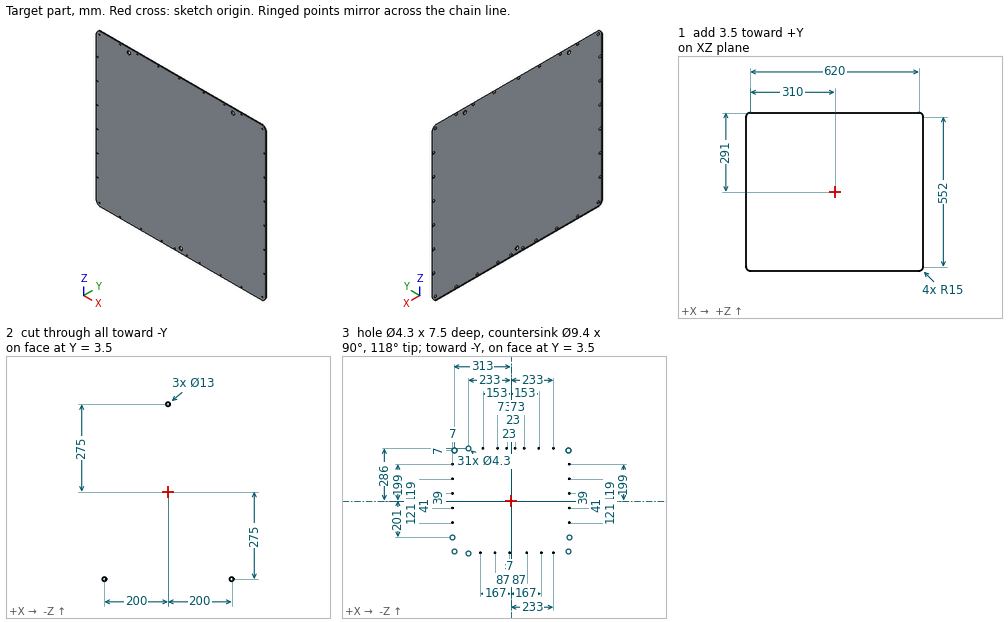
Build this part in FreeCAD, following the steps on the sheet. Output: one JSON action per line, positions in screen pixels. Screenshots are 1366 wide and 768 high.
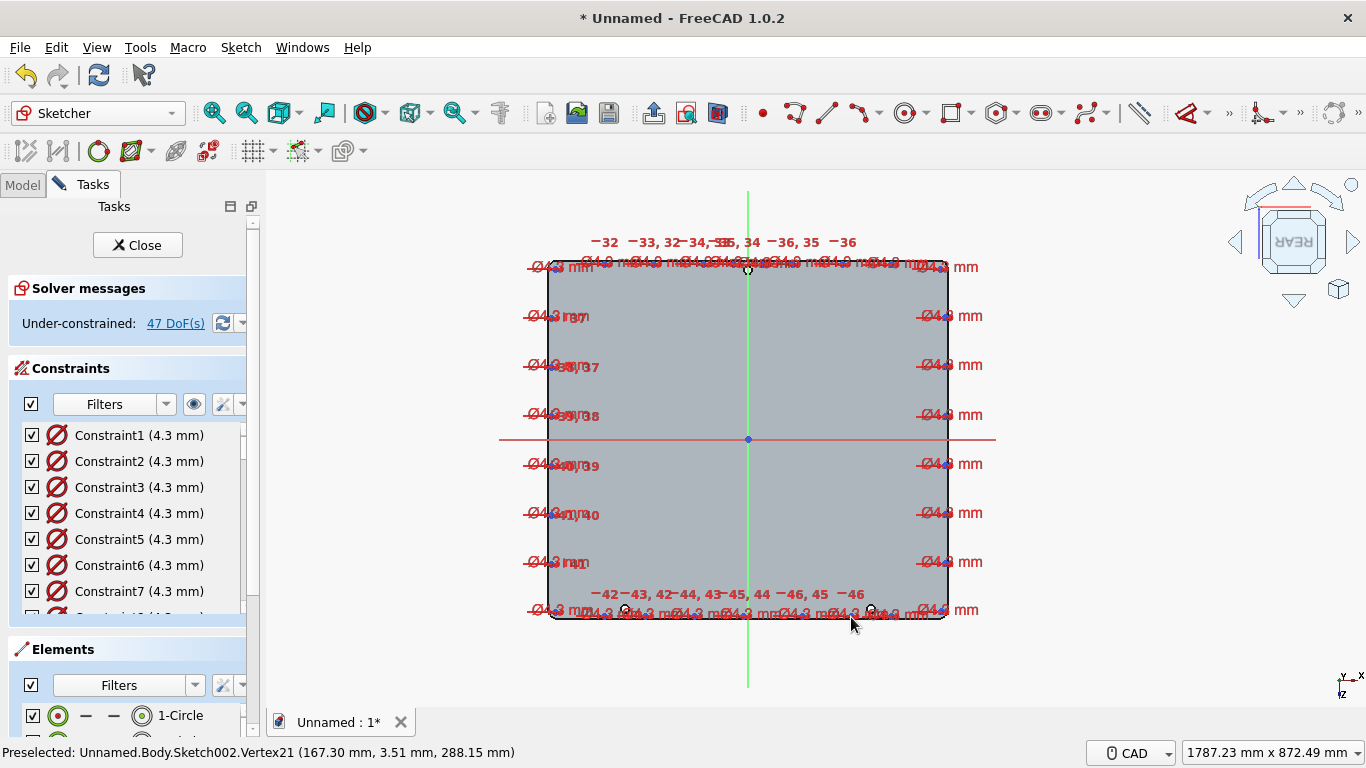
{"action": "left_click", "coordinate": [945, 564]}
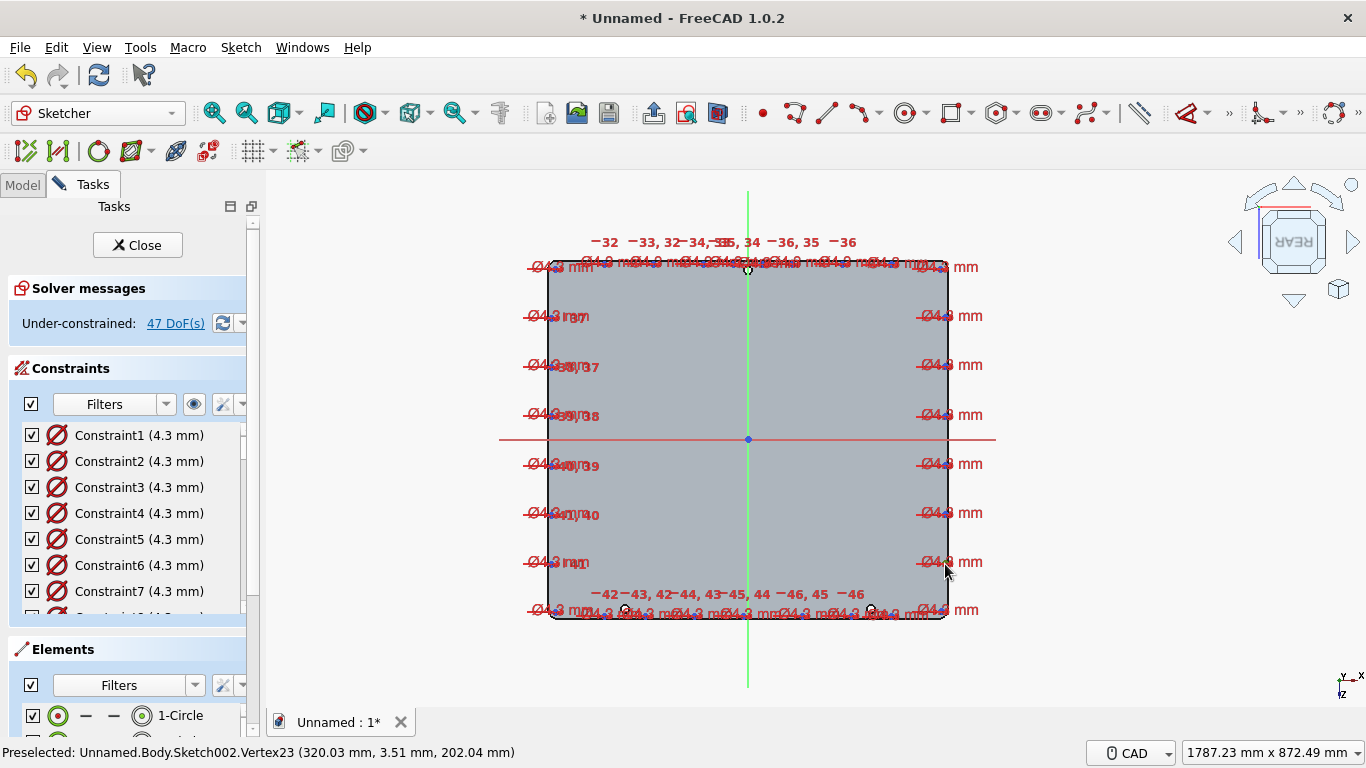
{"action": "left_click", "coordinate": [945, 515]}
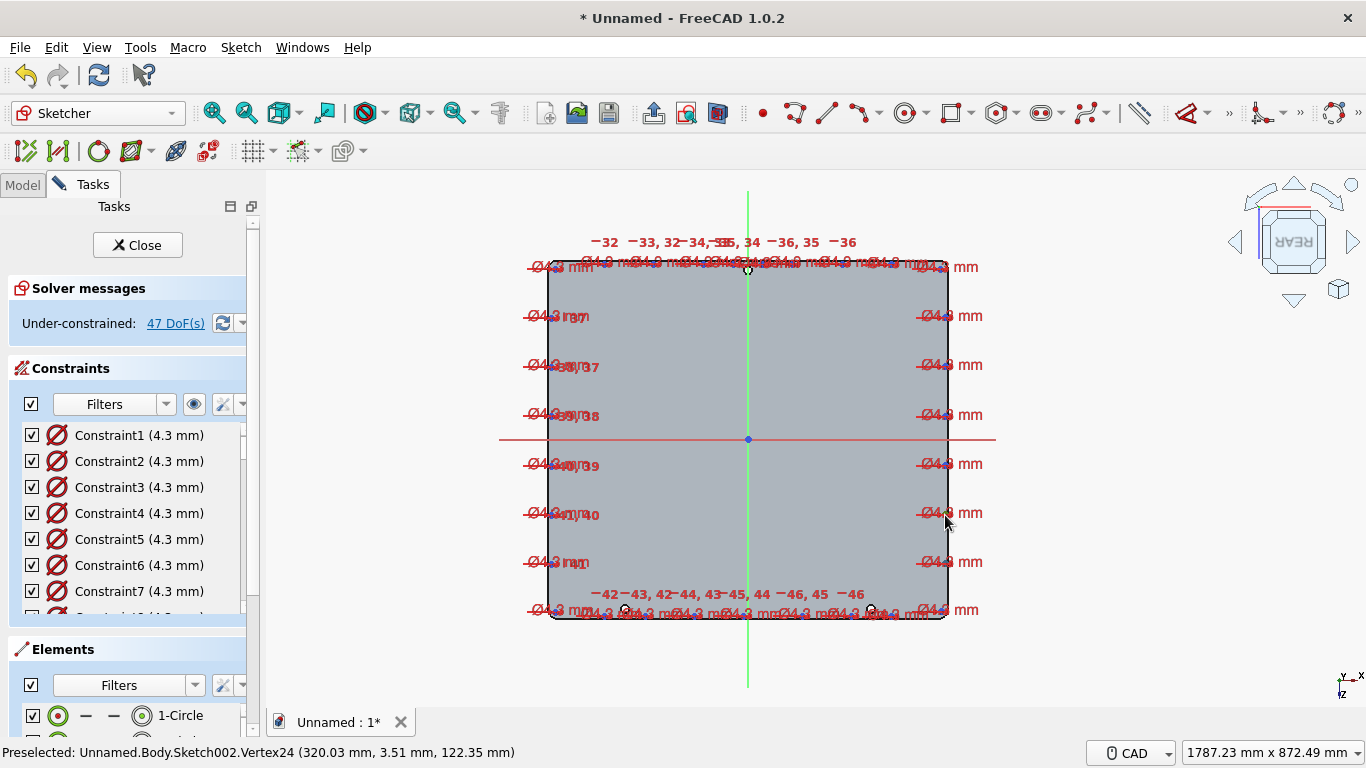
{"action": "key", "text": "v"}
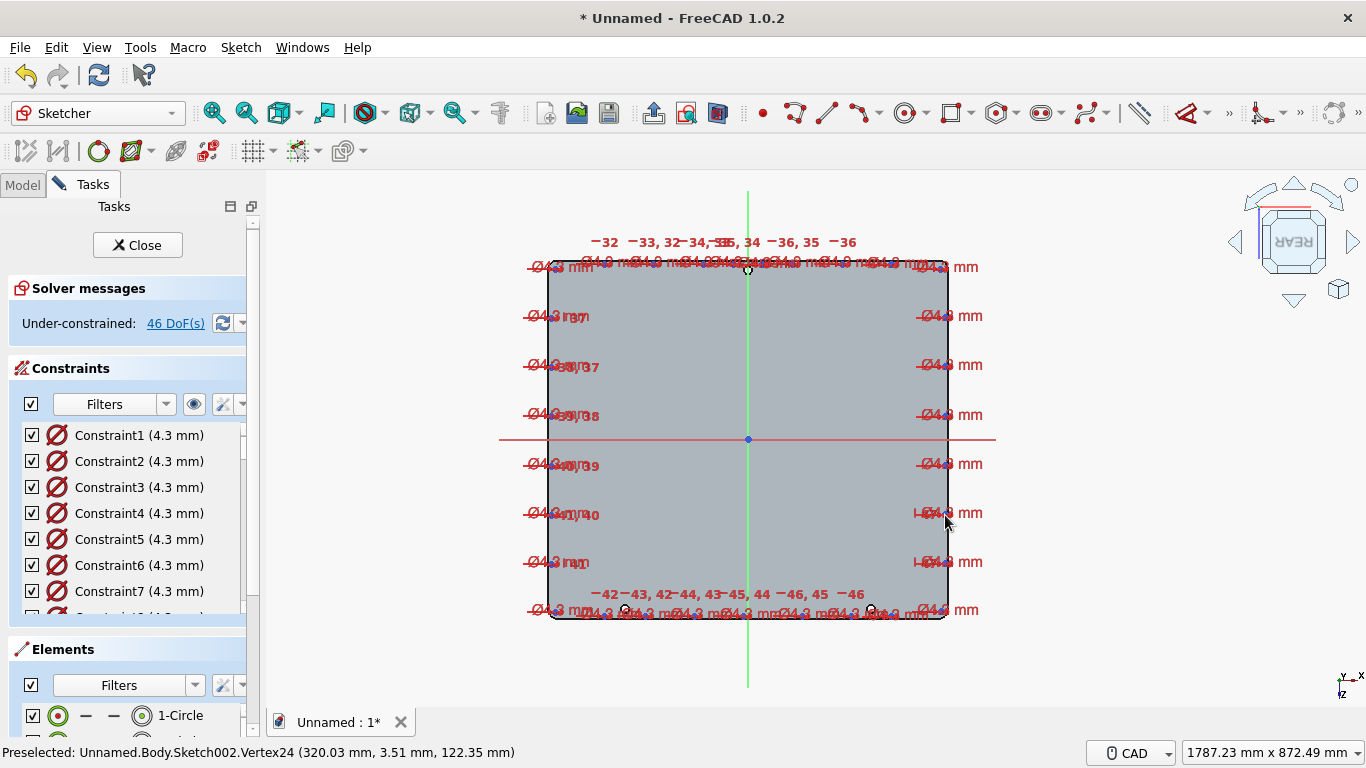
{"action": "left_click", "coordinate": [945, 515]}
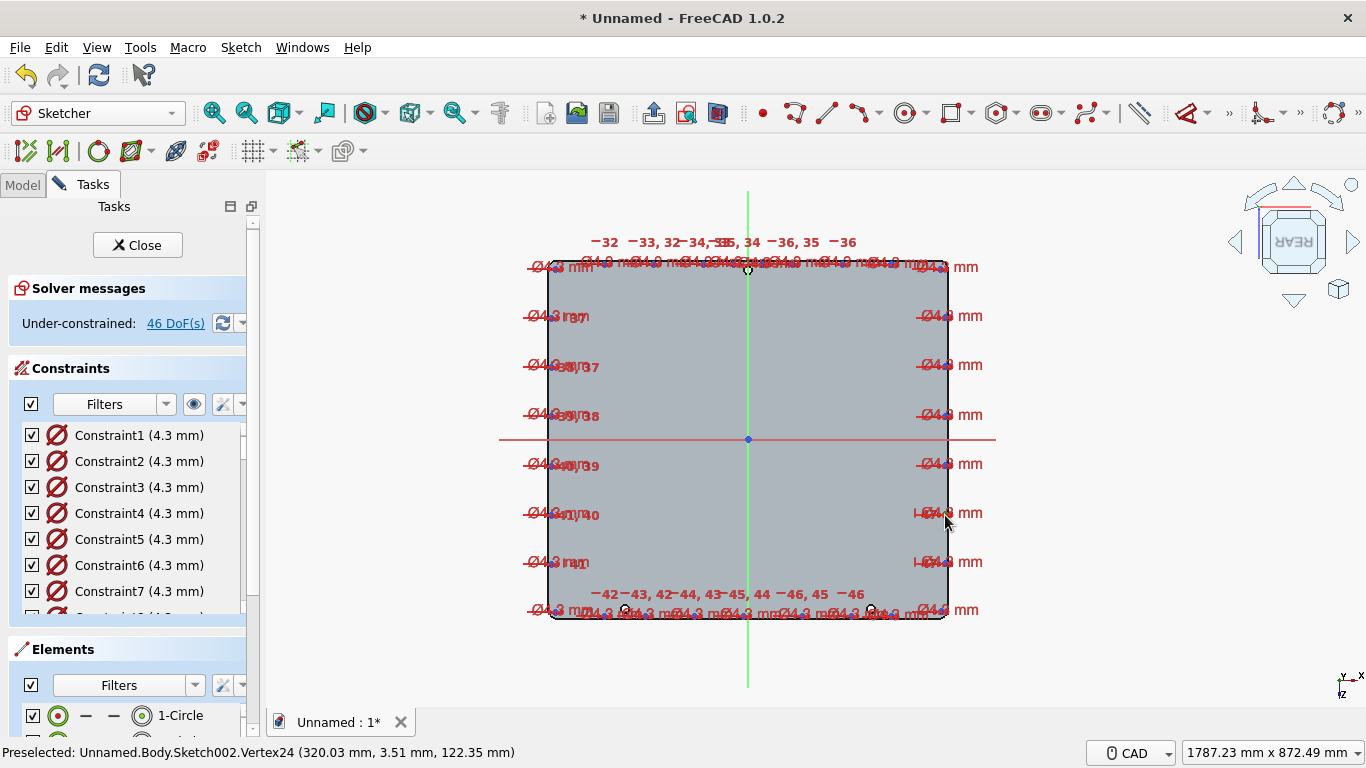
{"action": "left_click", "coordinate": [945, 466]}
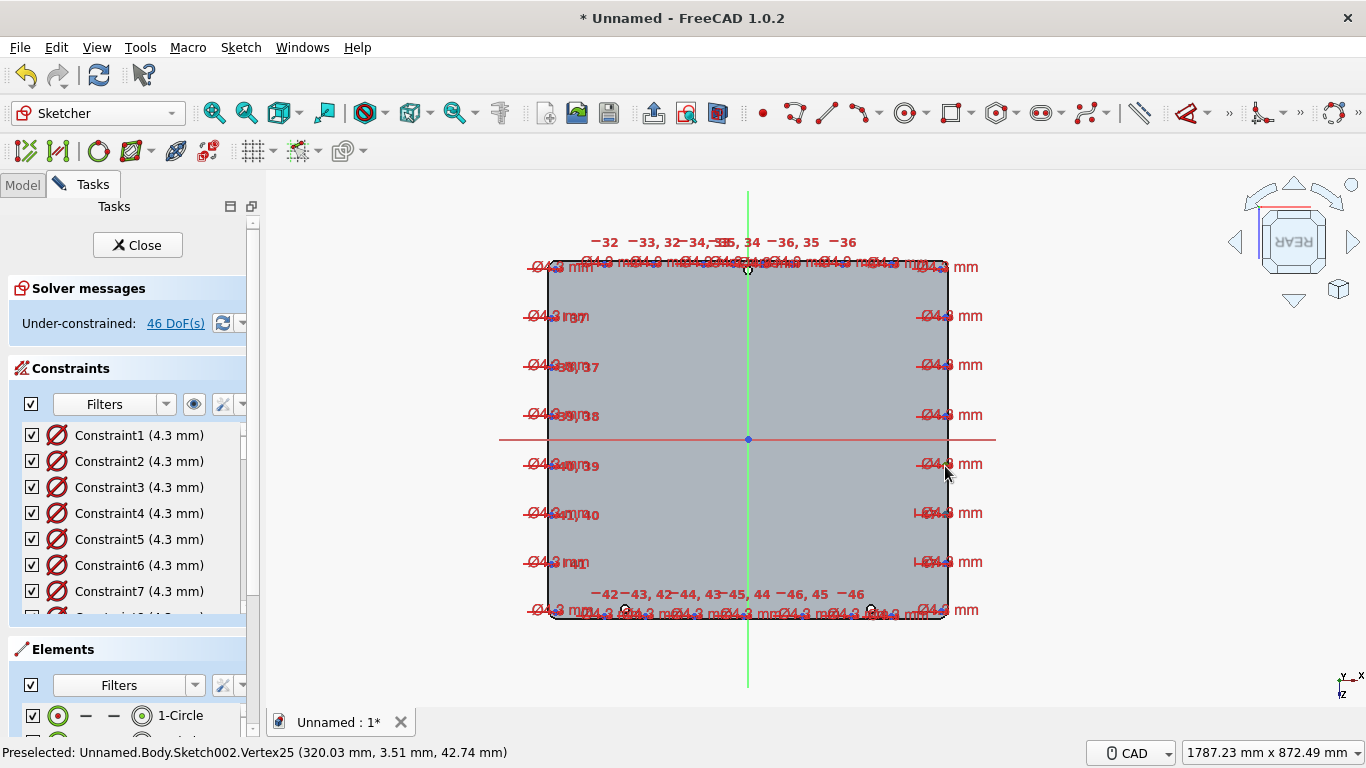
{"action": "key", "text": "v"}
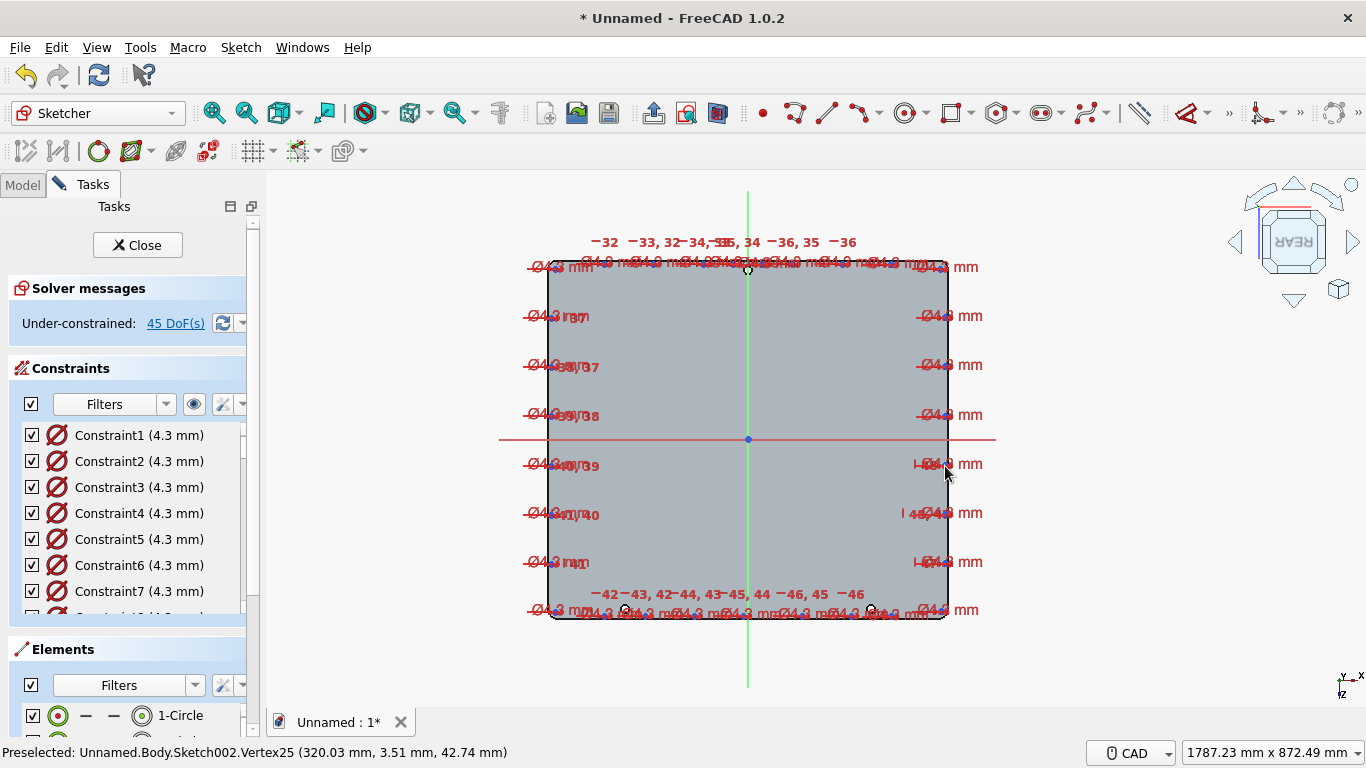
{"action": "left_click", "coordinate": [945, 466]}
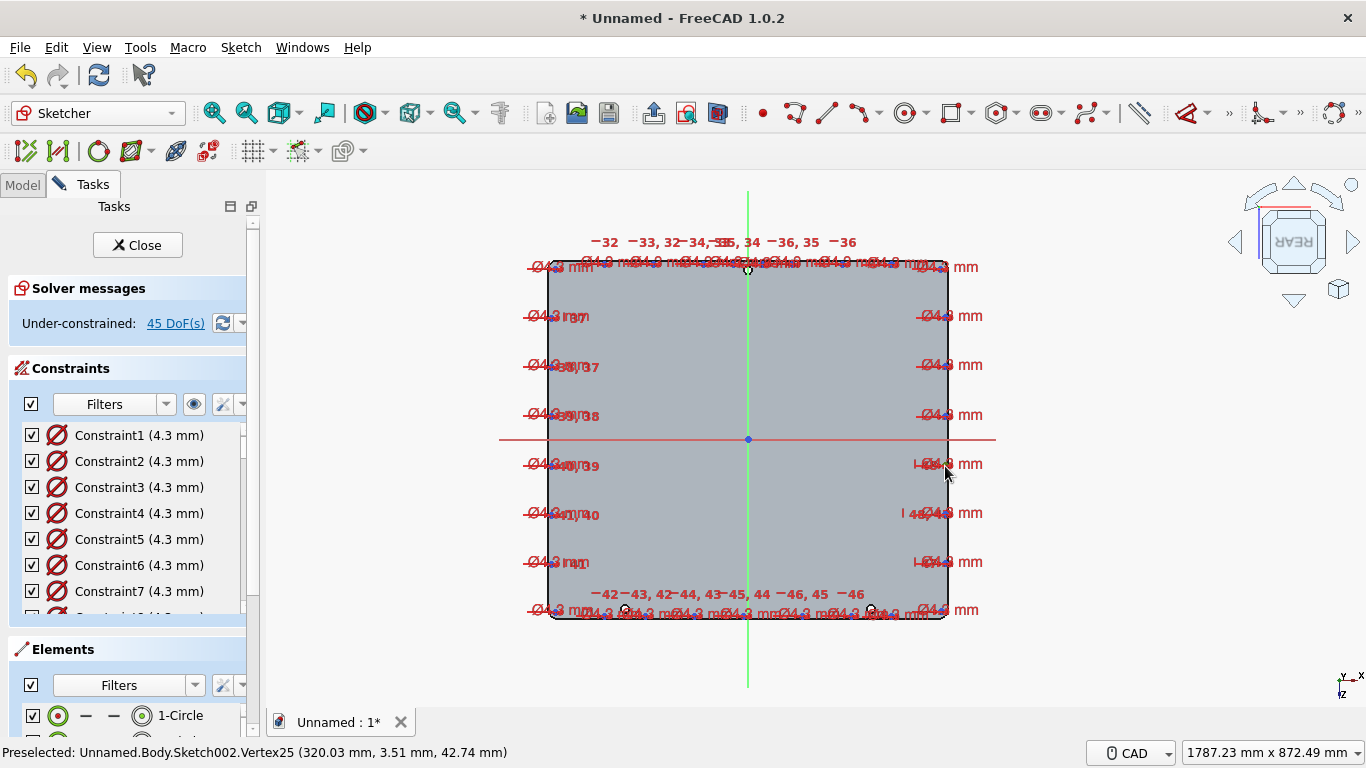
{"action": "left_click", "coordinate": [945, 417]}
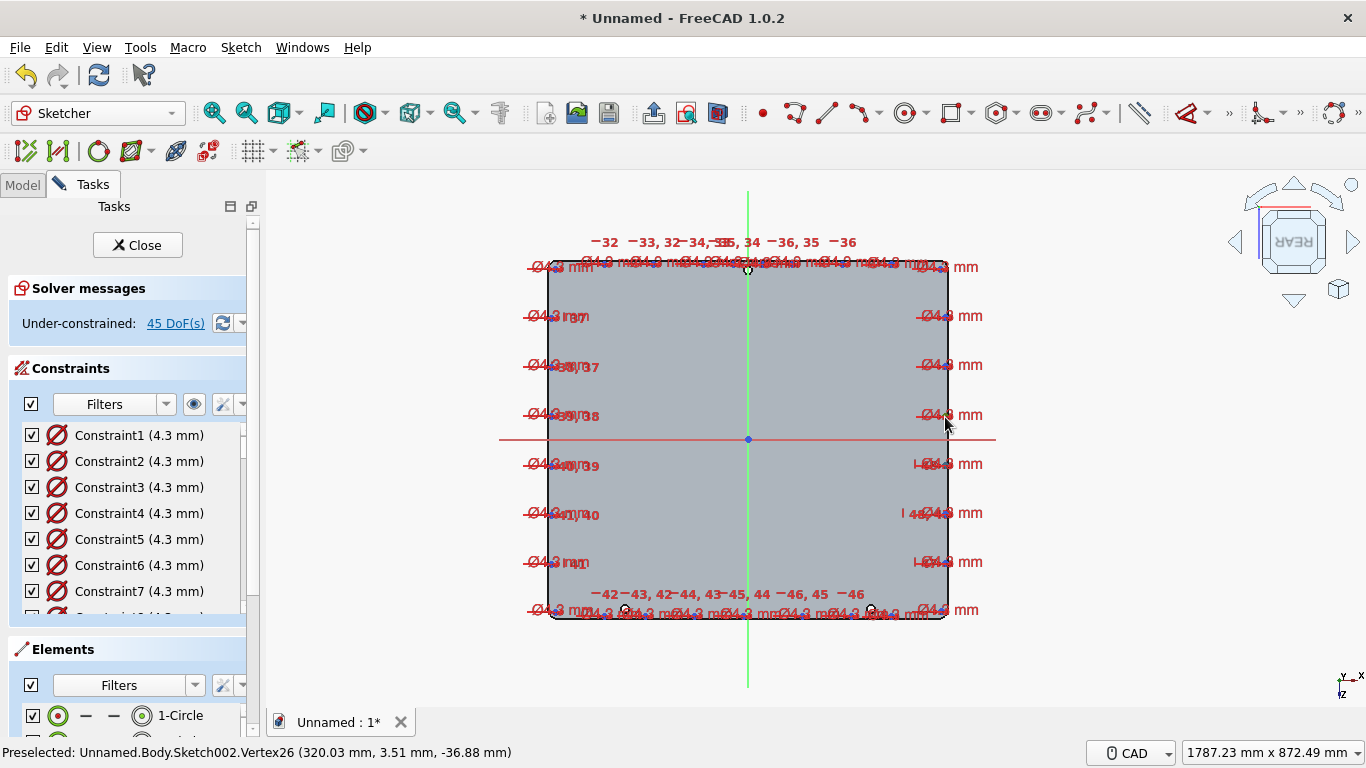
{"action": "key", "text": "v"}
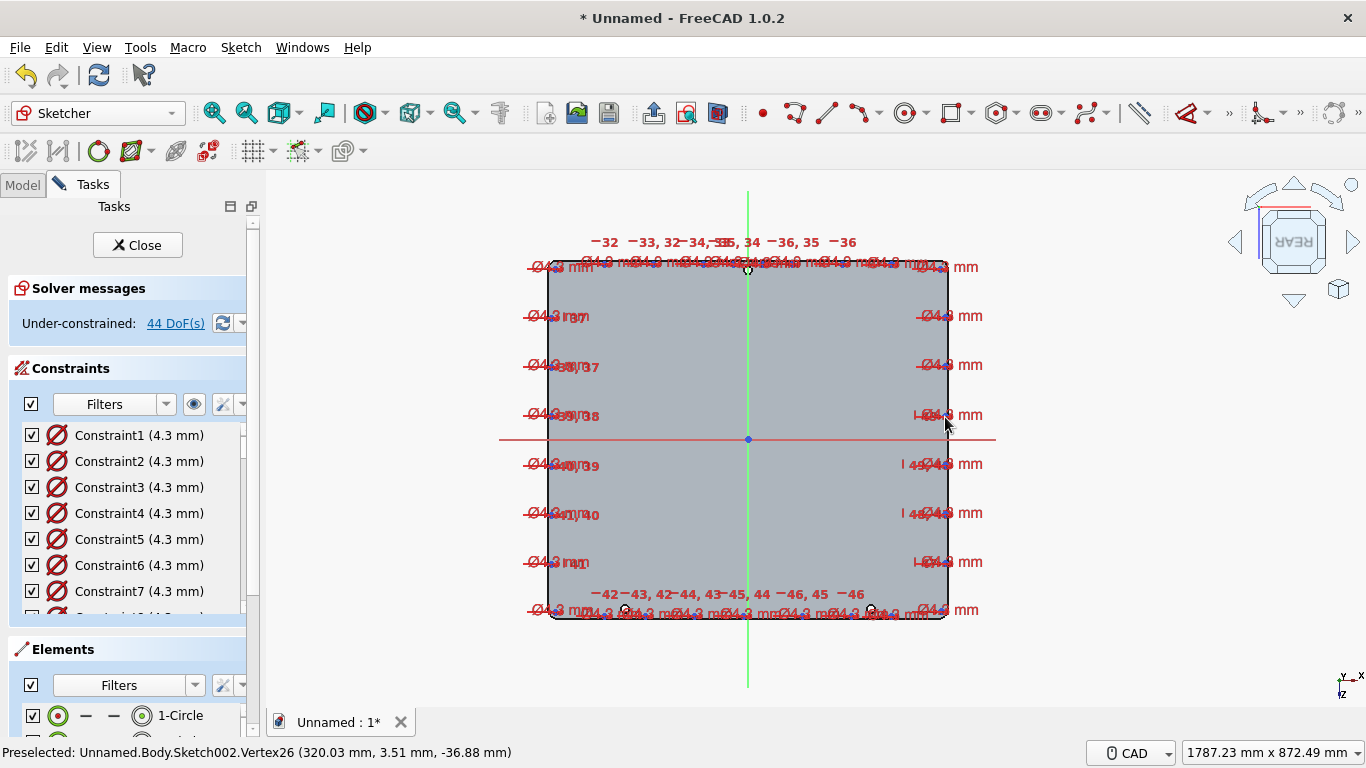
{"action": "left_click", "coordinate": [945, 417]}